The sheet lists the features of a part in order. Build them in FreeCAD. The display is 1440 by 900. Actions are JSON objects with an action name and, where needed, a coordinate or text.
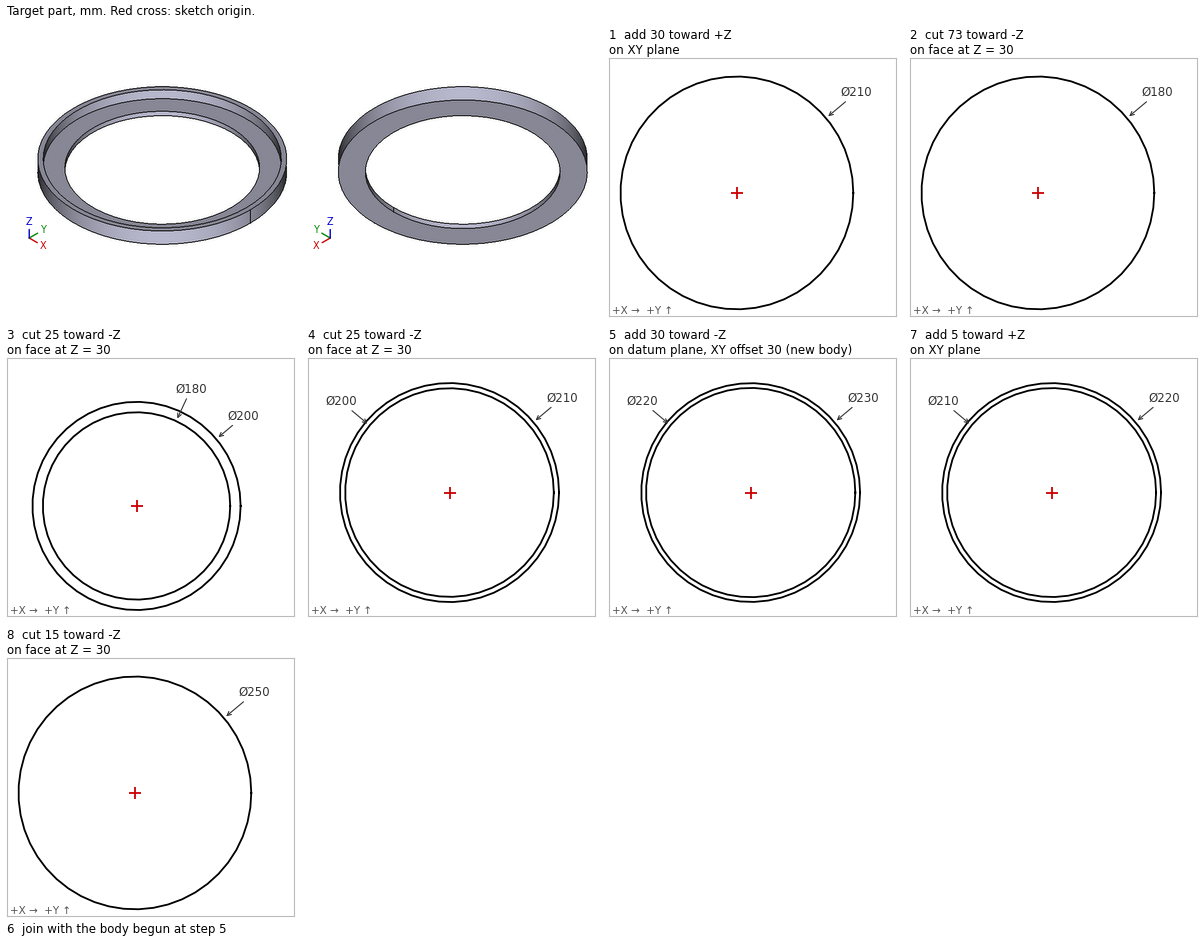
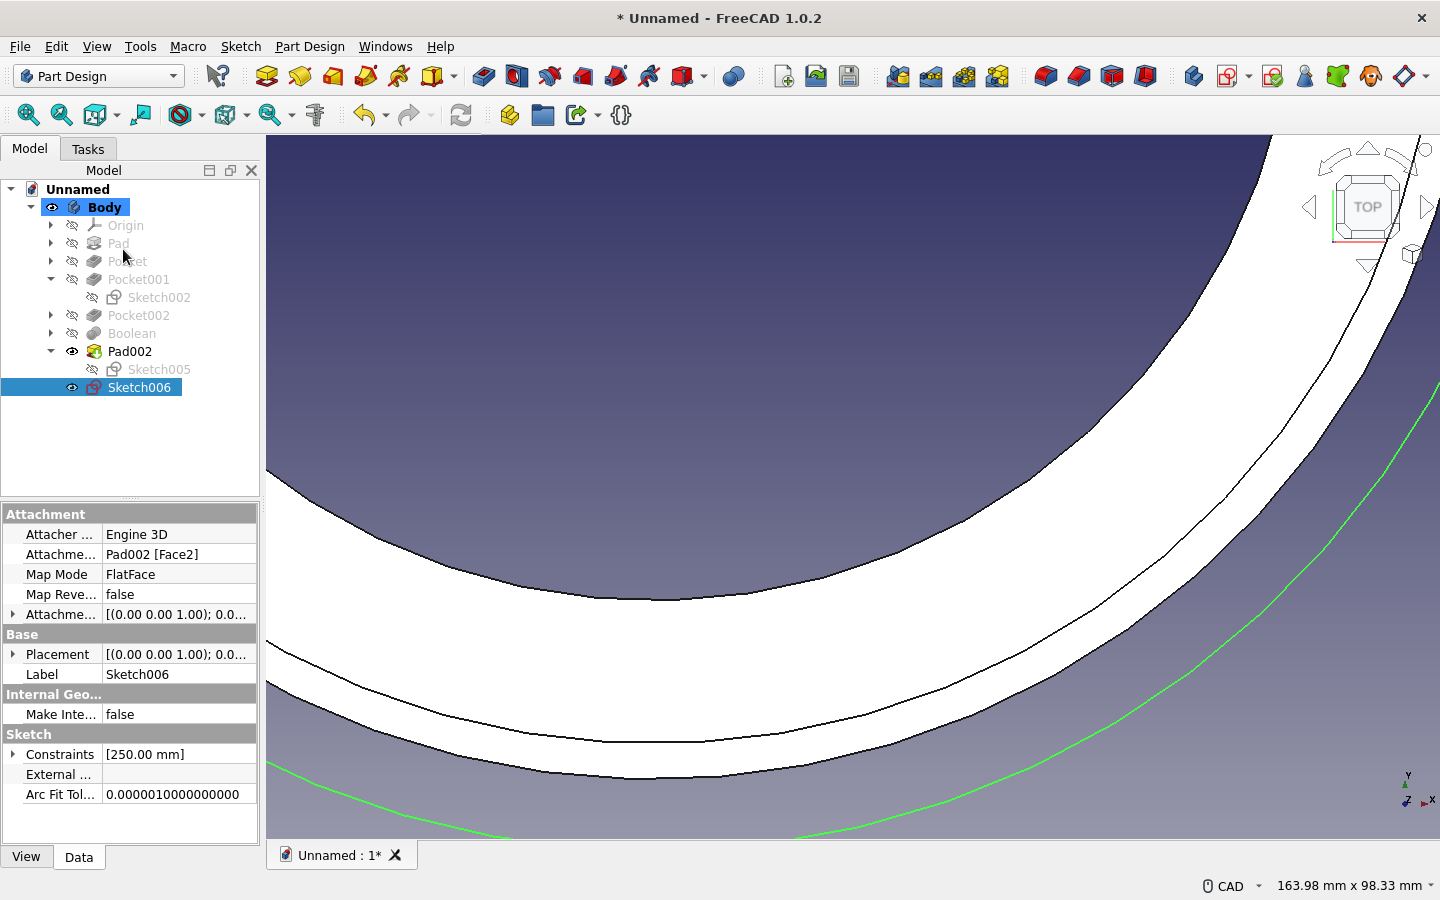
{"action": "left_click", "coordinate": [484, 76]}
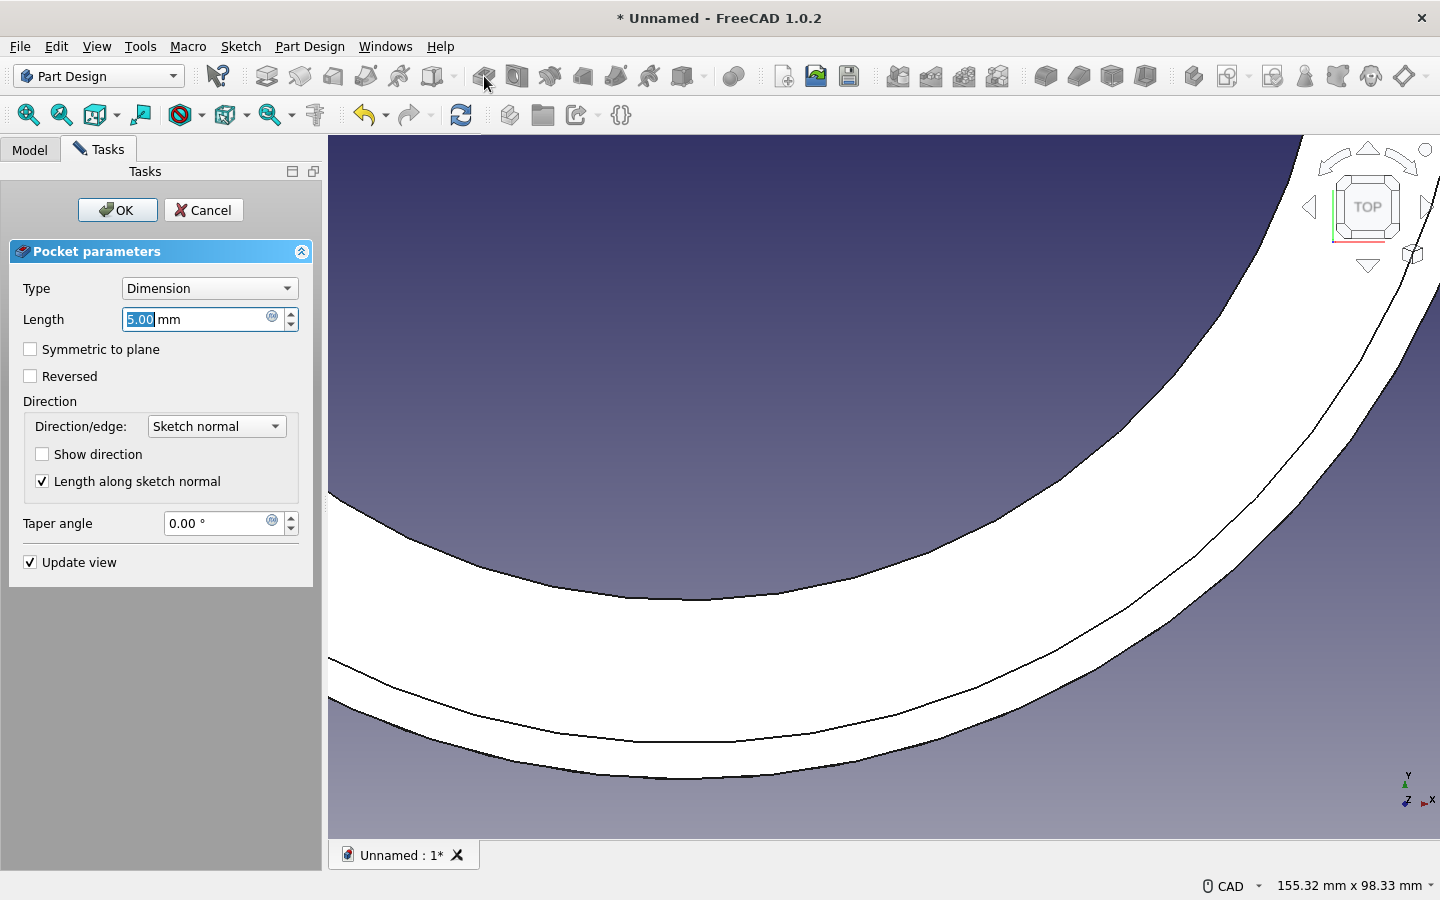
{"action": "type", "text": "15"}
{"action": "key", "text": "Tab"}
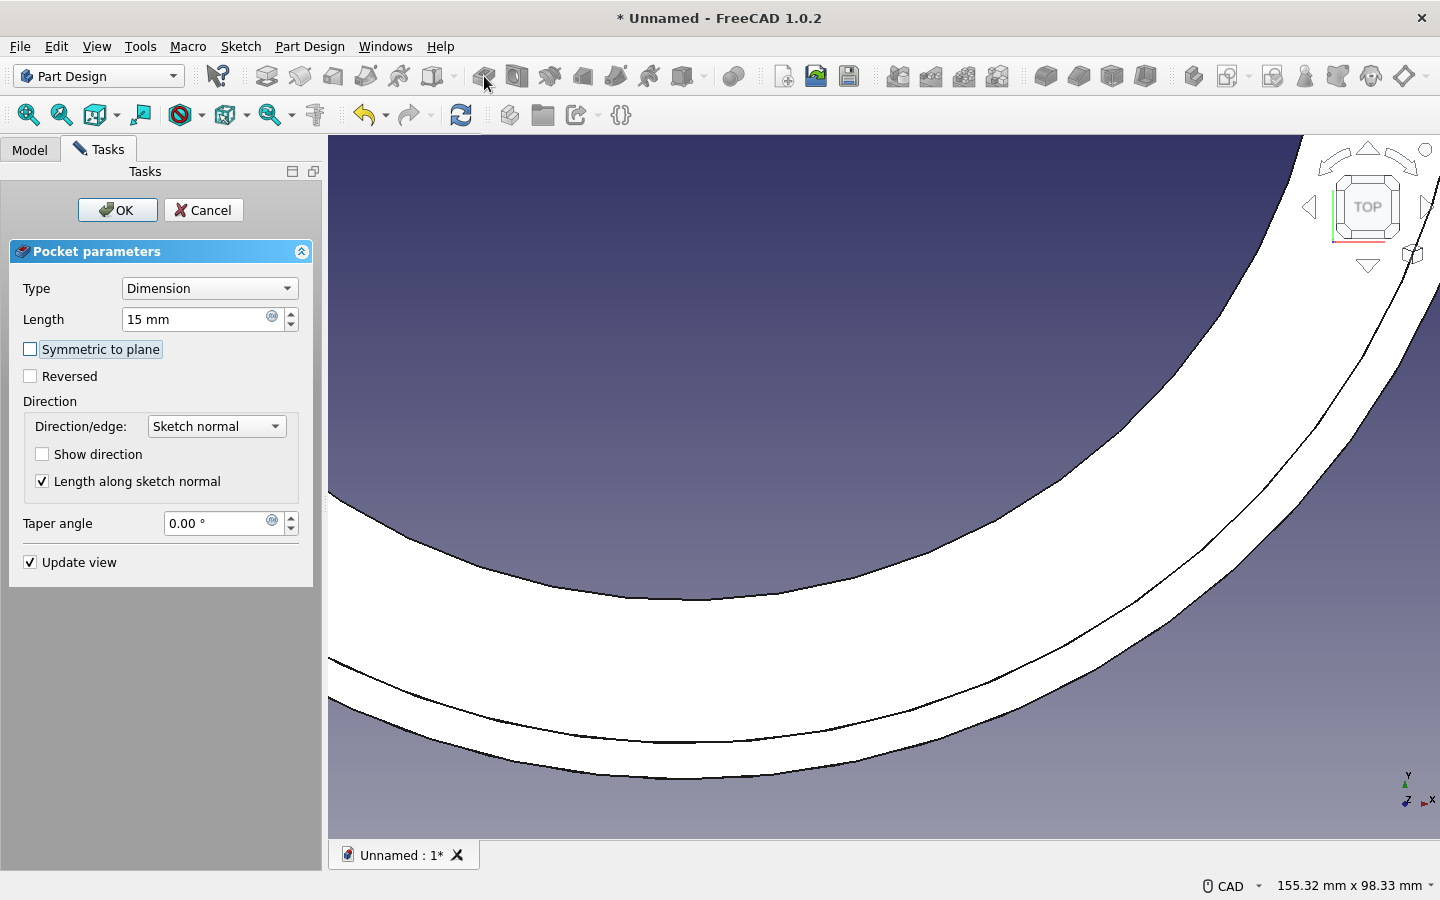
{"action": "left_click", "coordinate": [118, 210]}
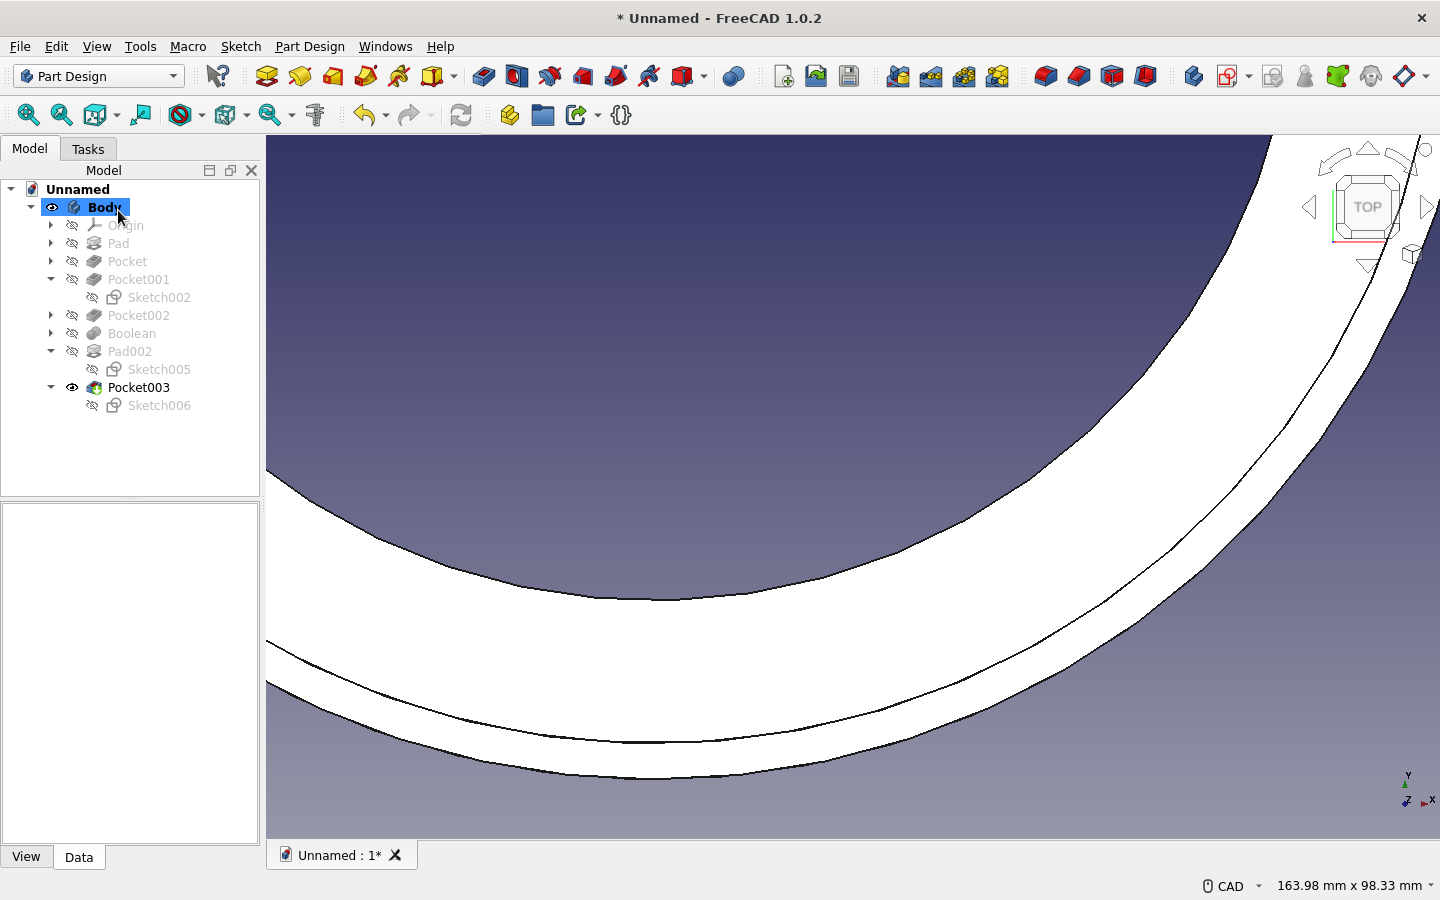
{"action": "key", "text": "0"}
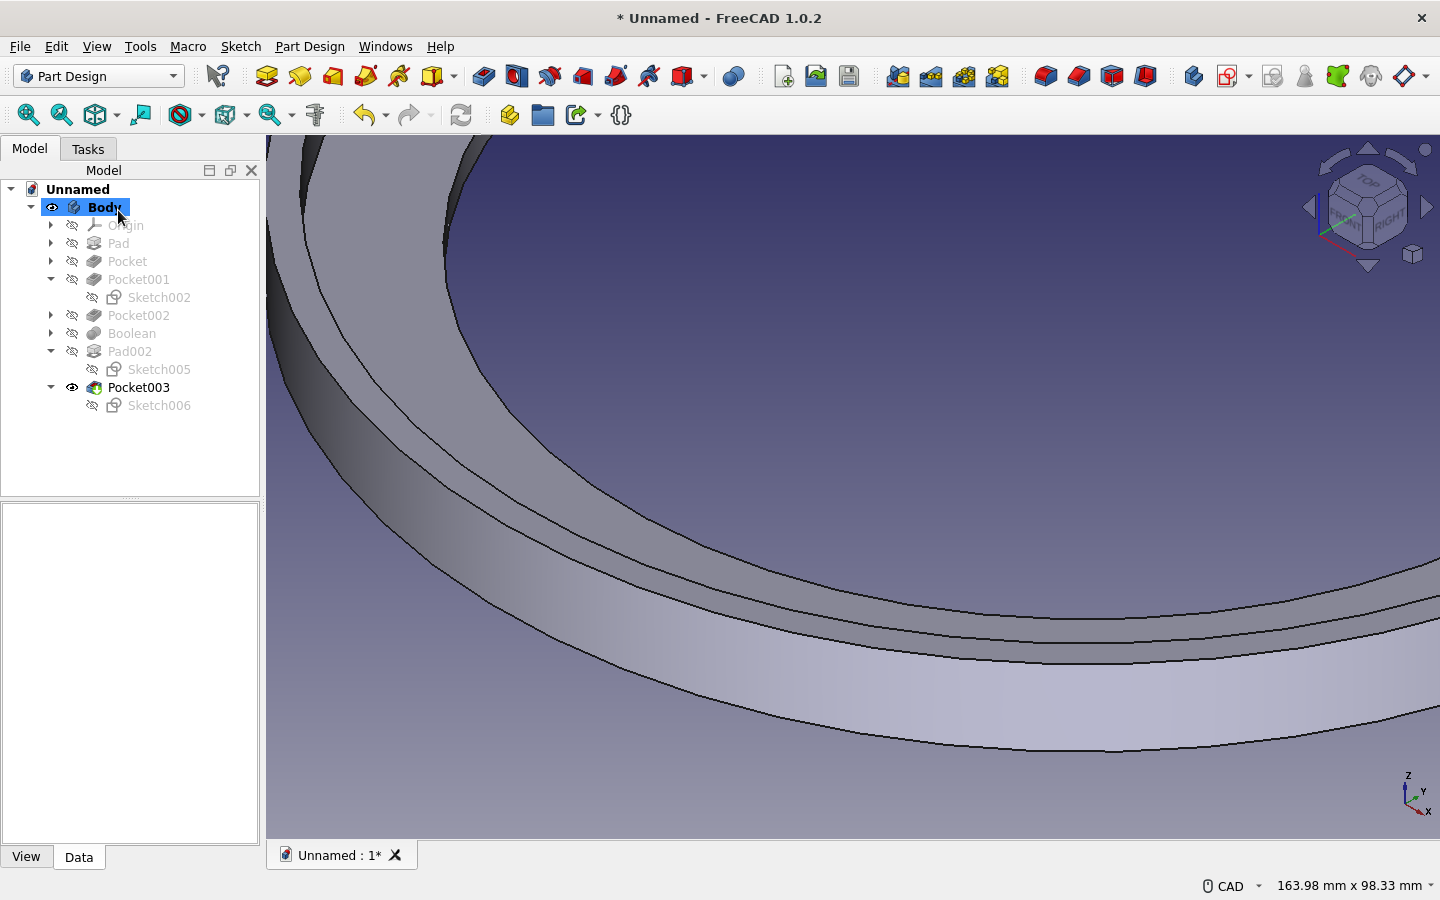
{"action": "left_click", "coordinate": [29, 116]}